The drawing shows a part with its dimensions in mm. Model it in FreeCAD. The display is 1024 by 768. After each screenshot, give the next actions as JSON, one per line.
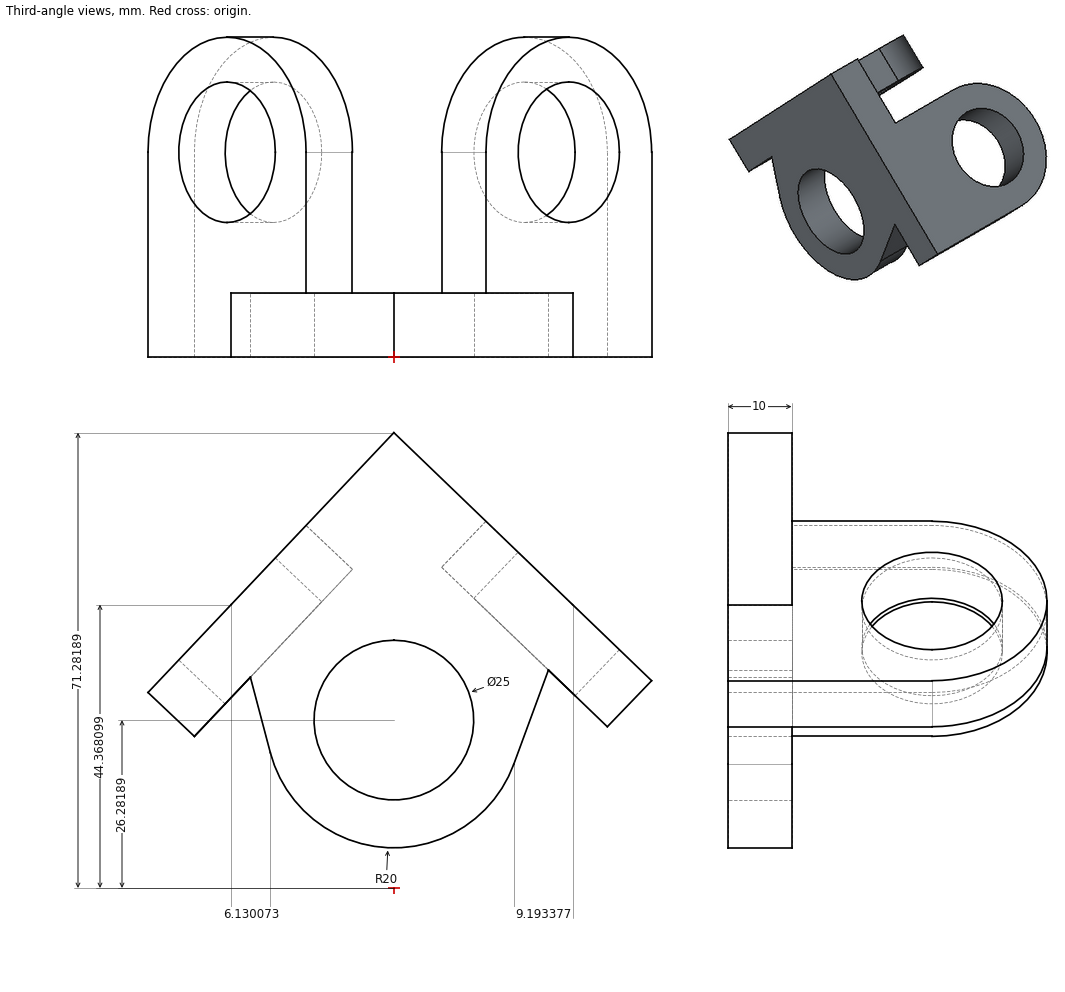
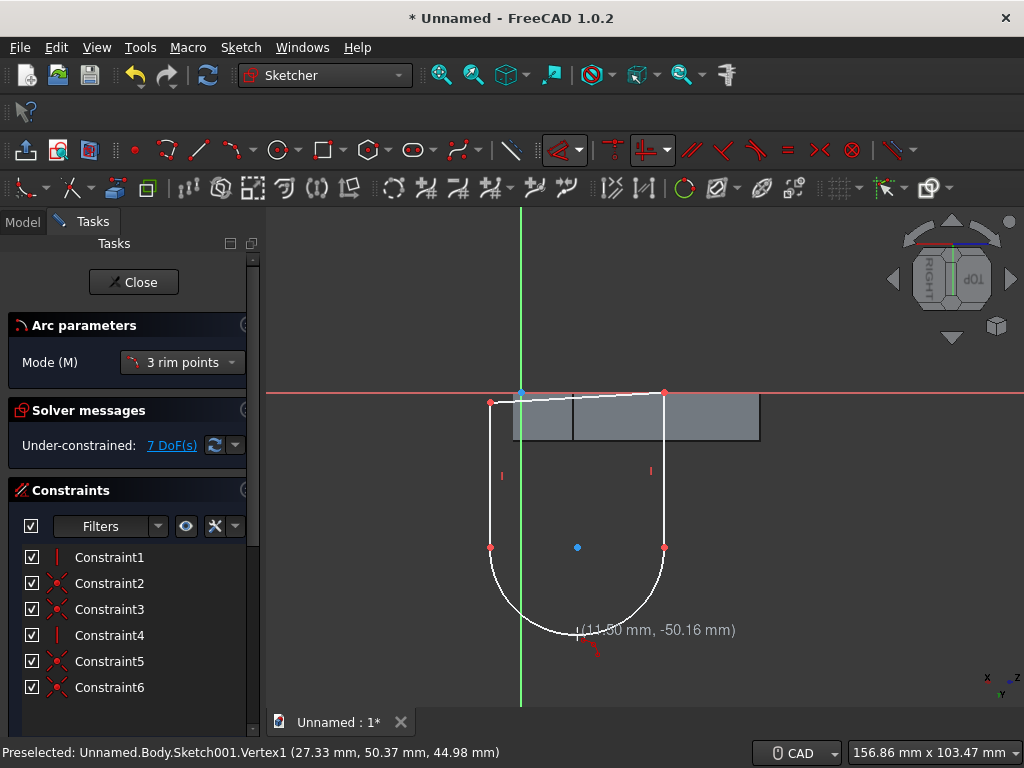
{"action": "left_click", "coordinate": [278, 150]}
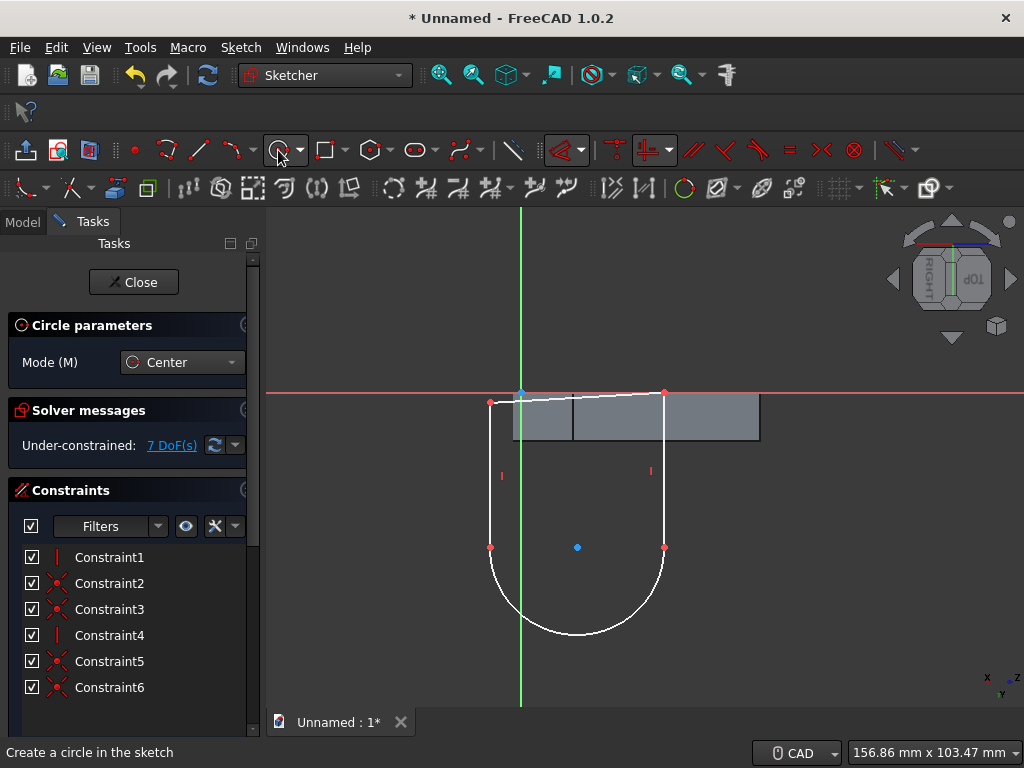
{"action": "left_click", "coordinate": [577, 547]}
{"action": "mouse_move", "coordinate": [614, 510]}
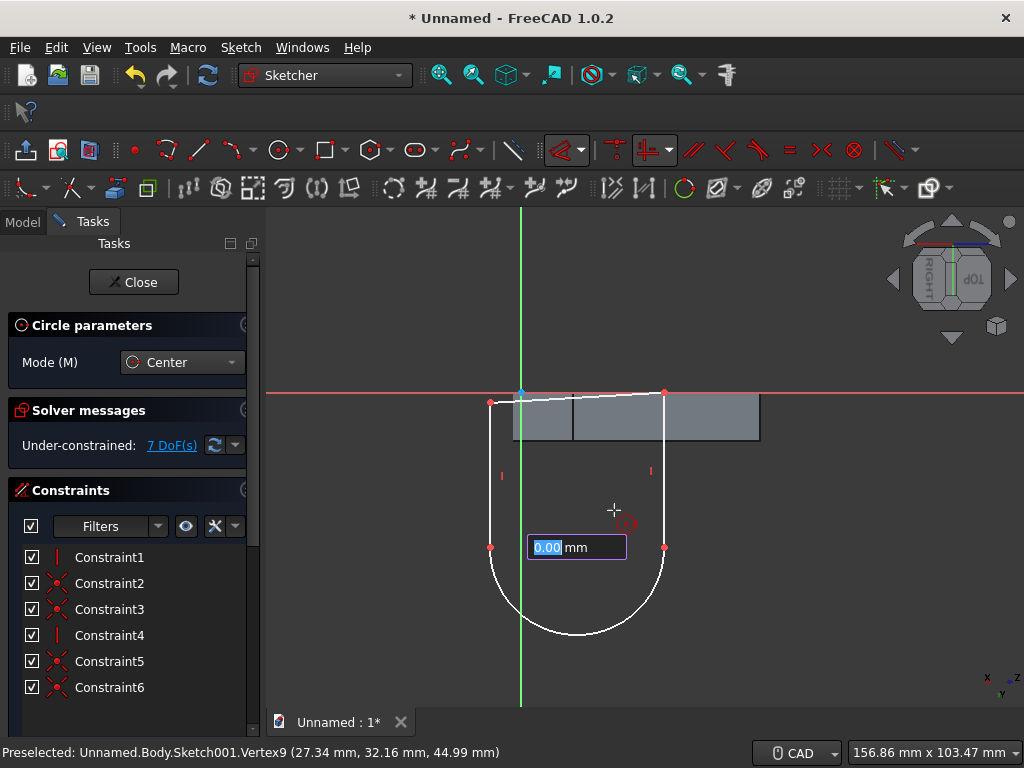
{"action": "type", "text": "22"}
{"action": "key", "text": "Return"}
{"action": "key", "text": "Escape"}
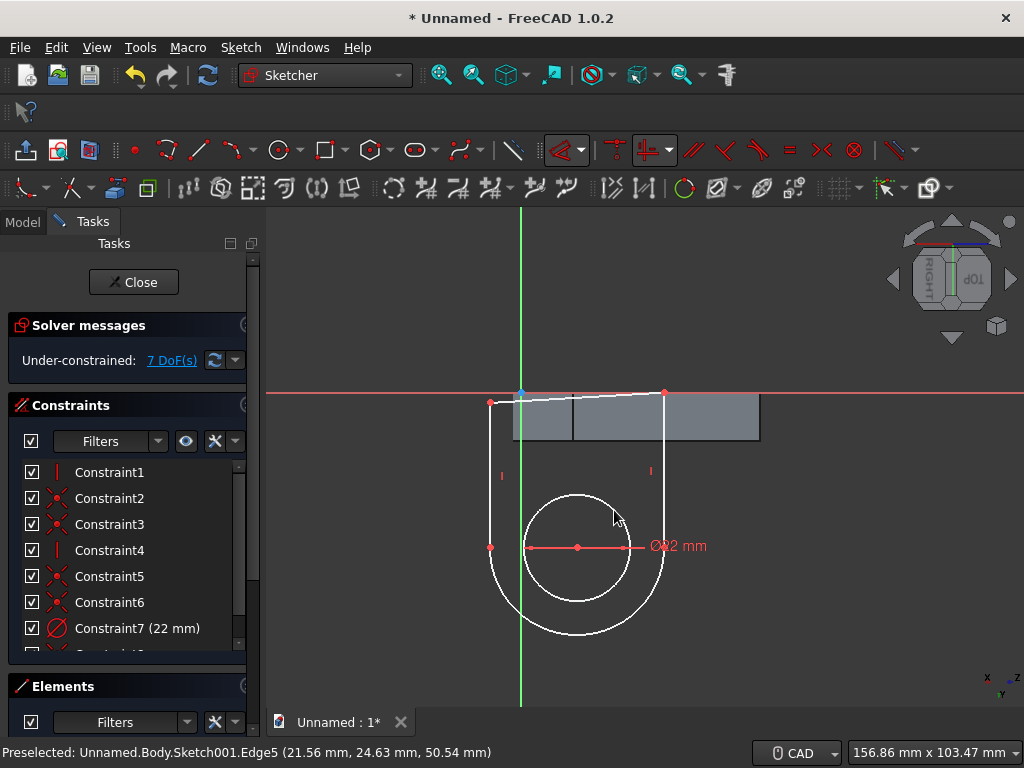
{"action": "left_click", "coordinate": [664, 501]}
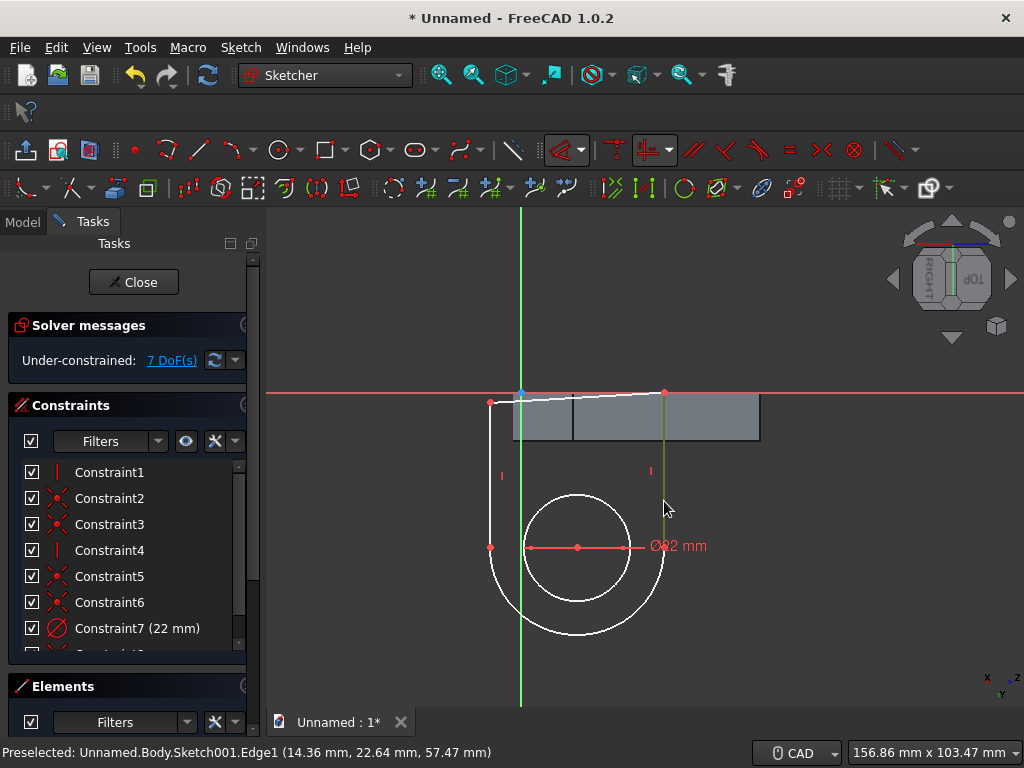
{"action": "left_click", "coordinate": [628, 618]}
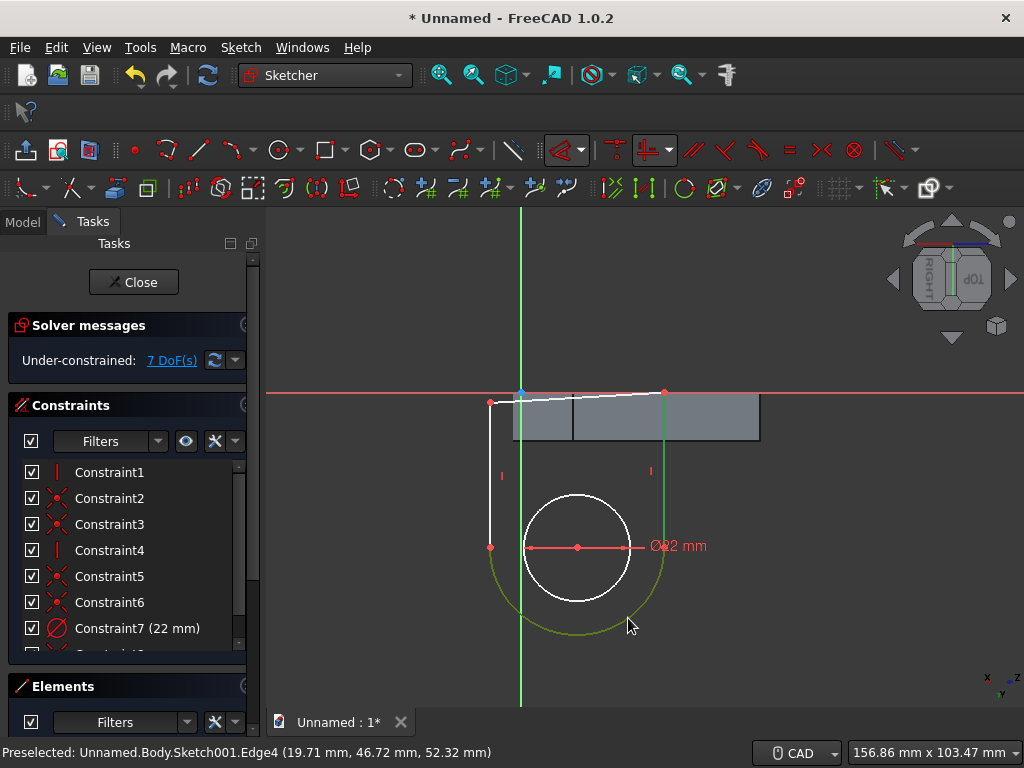
{"action": "left_click", "coordinate": [758, 150]}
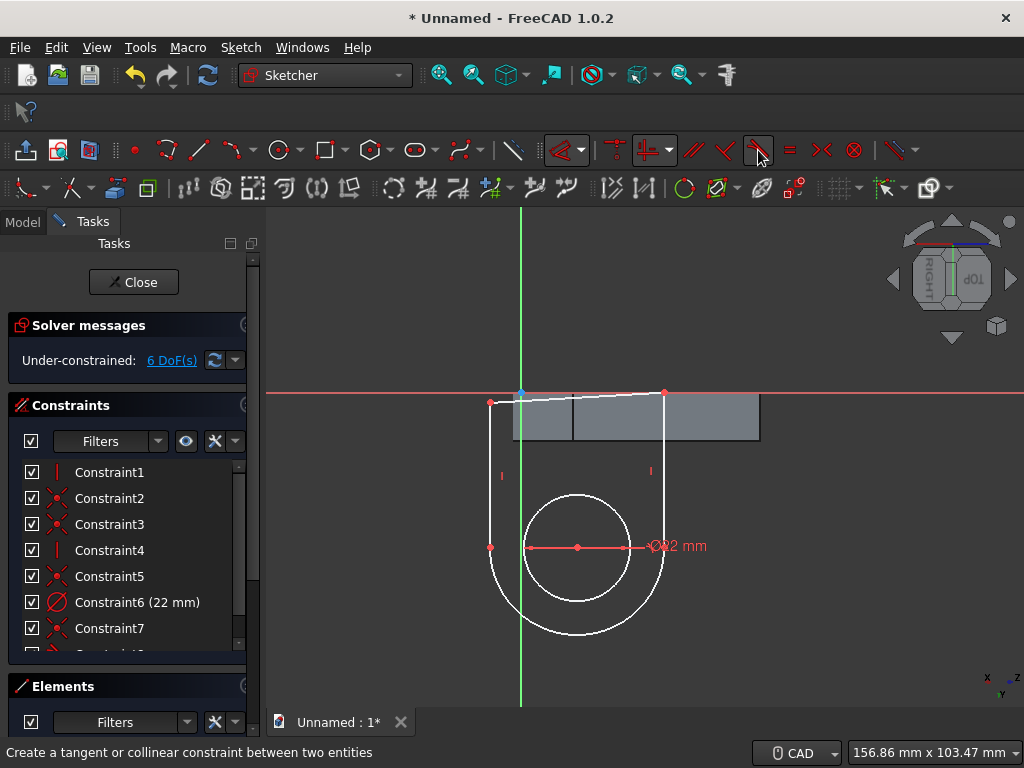
{"action": "left_click", "coordinate": [490, 447]}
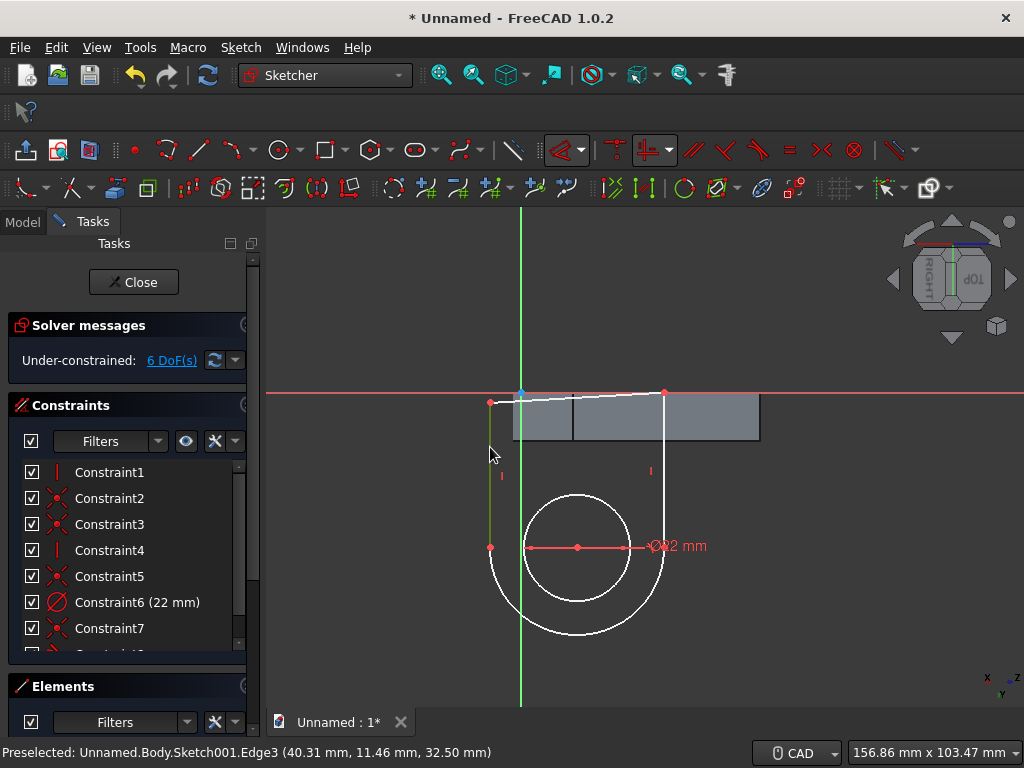
{"action": "left_click", "coordinate": [628, 618]}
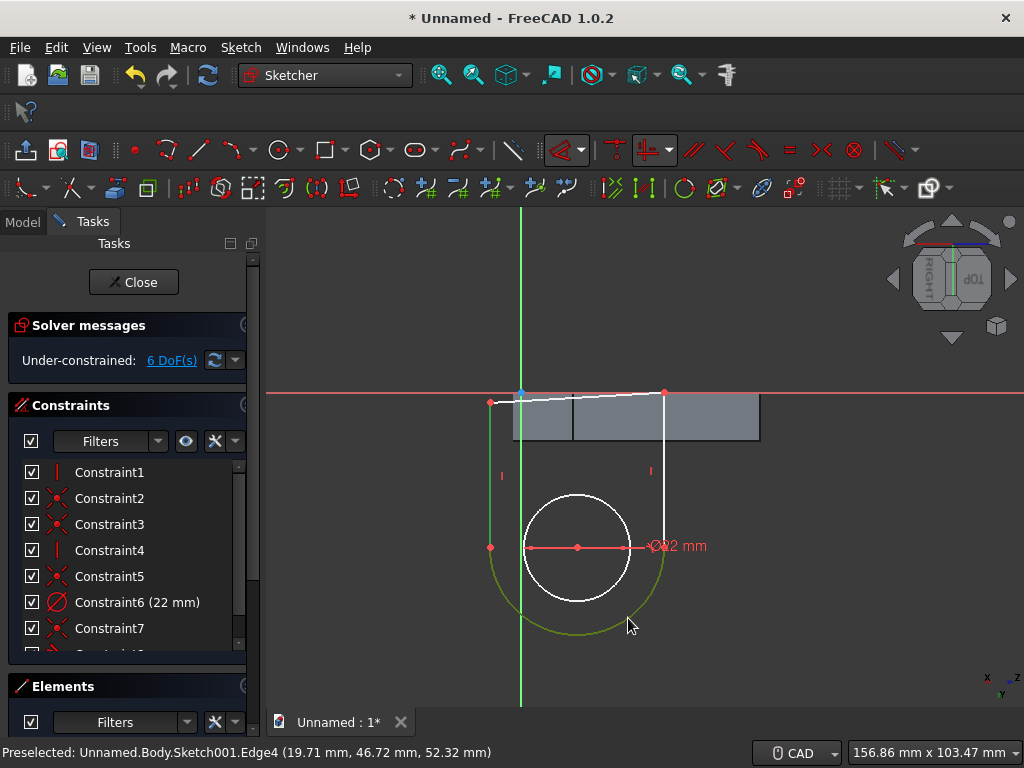
{"action": "left_click", "coordinate": [758, 150]}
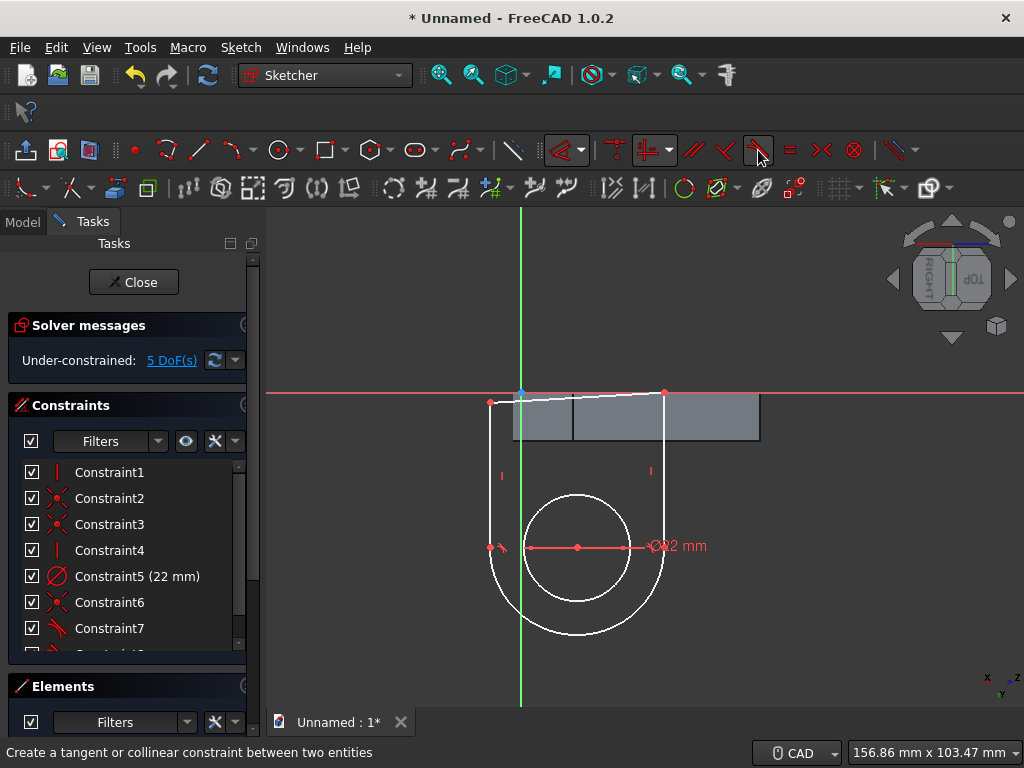
{"action": "left_click", "coordinate": [612, 396]}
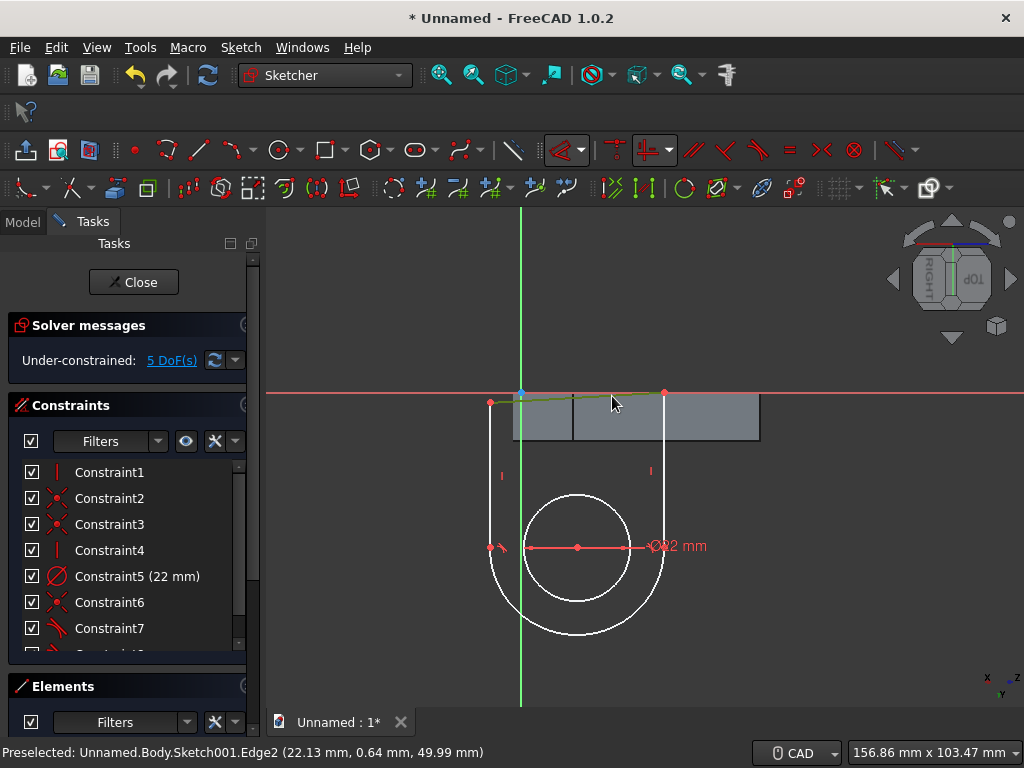
{"action": "left_click", "coordinate": [672, 150]}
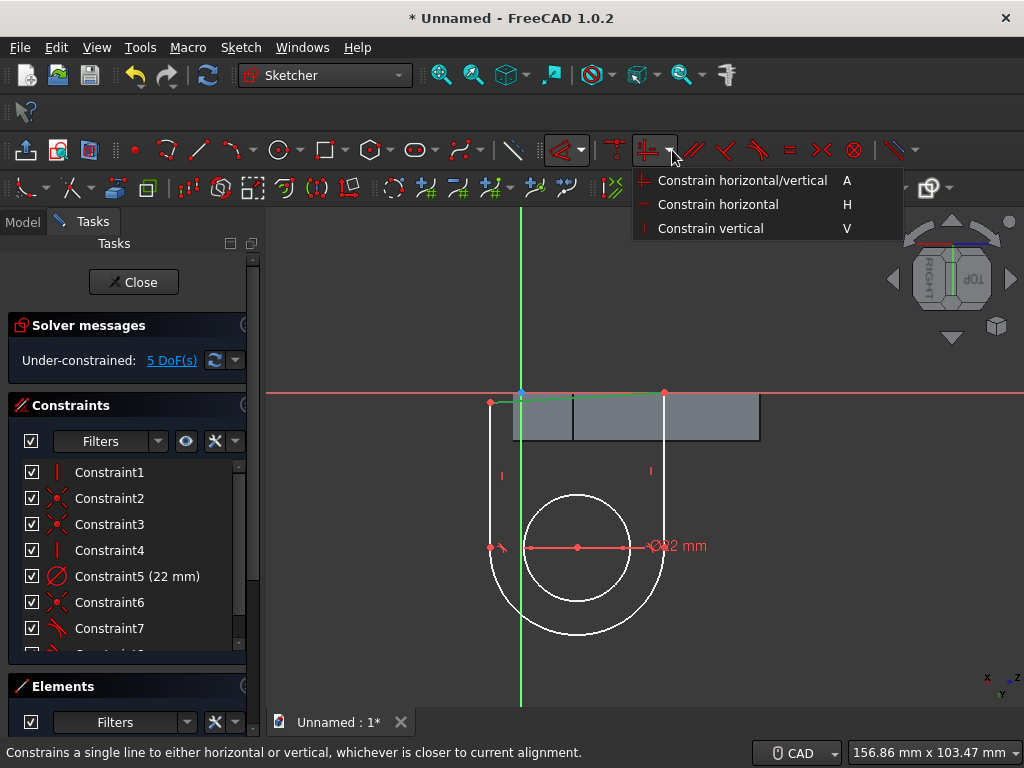
{"action": "left_click", "coordinate": [768, 204]}